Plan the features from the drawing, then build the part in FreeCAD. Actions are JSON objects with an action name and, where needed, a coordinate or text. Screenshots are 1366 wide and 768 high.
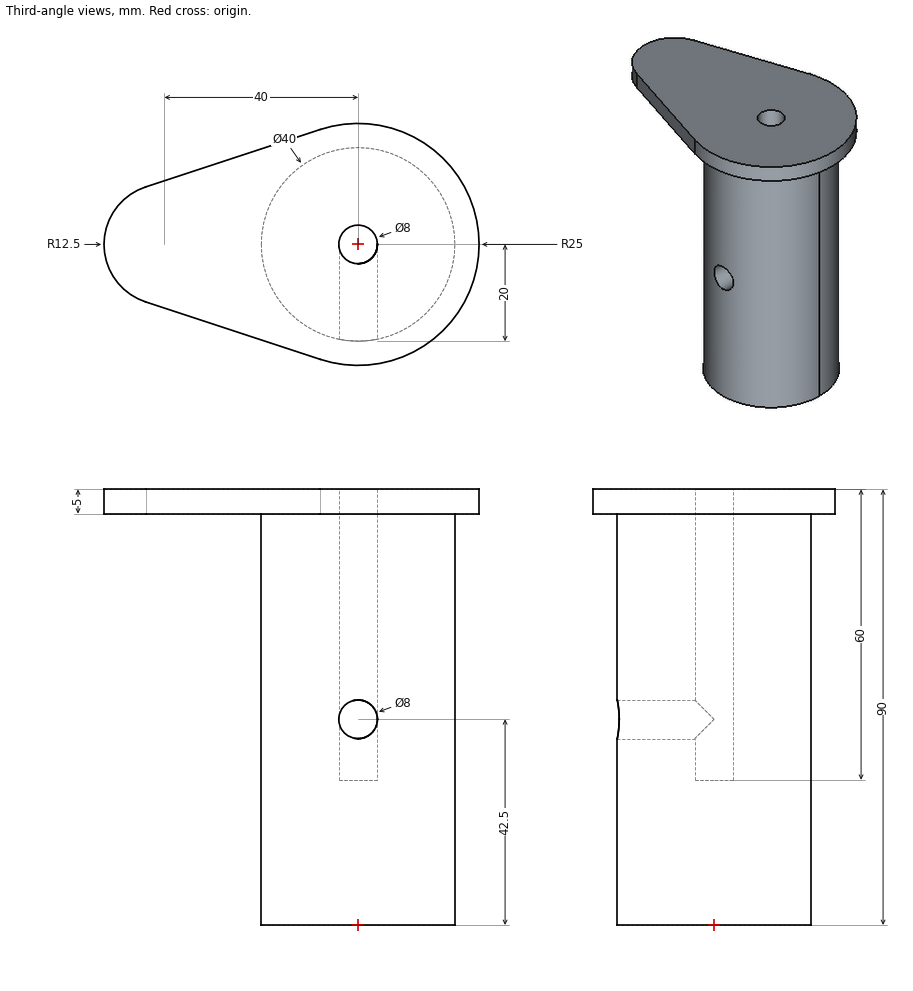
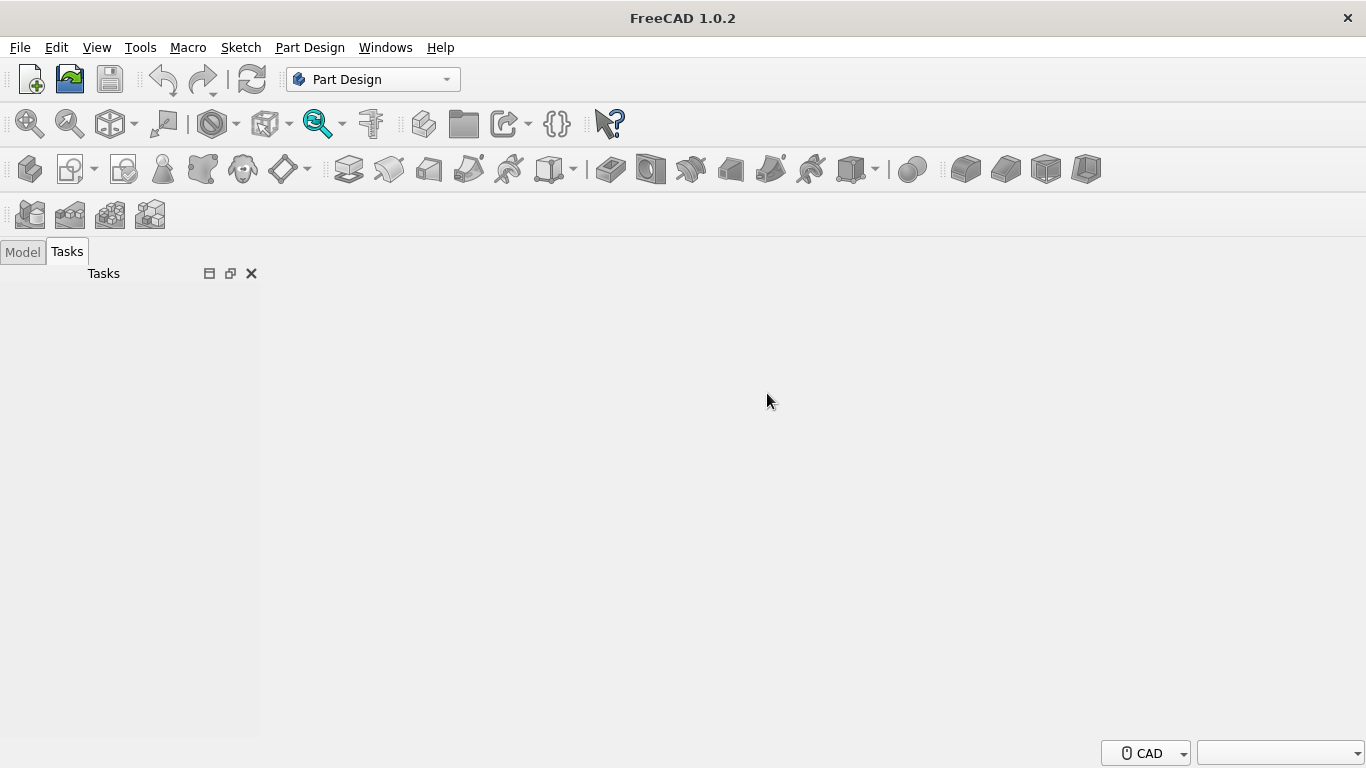
{"action": "key", "text": "ctrl+n"}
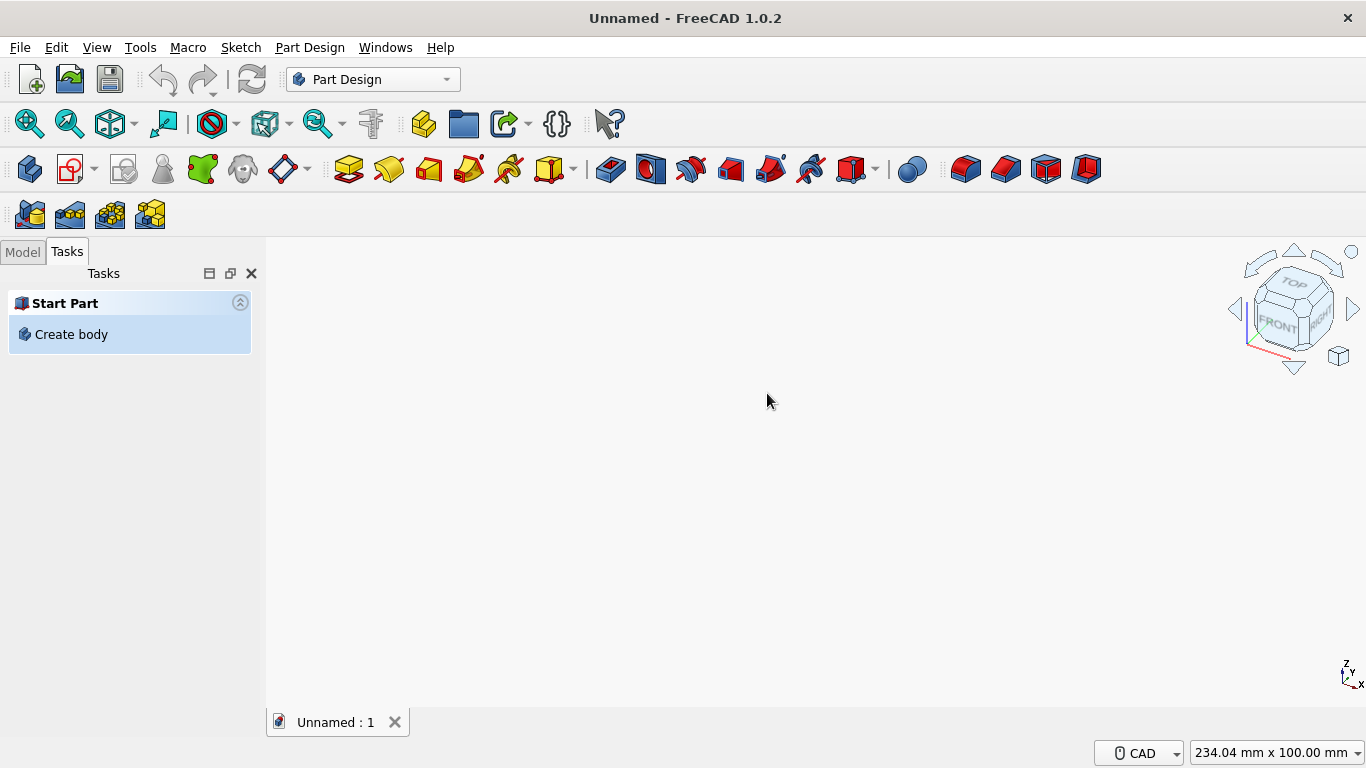
{"action": "left_click", "coordinate": [70, 170]}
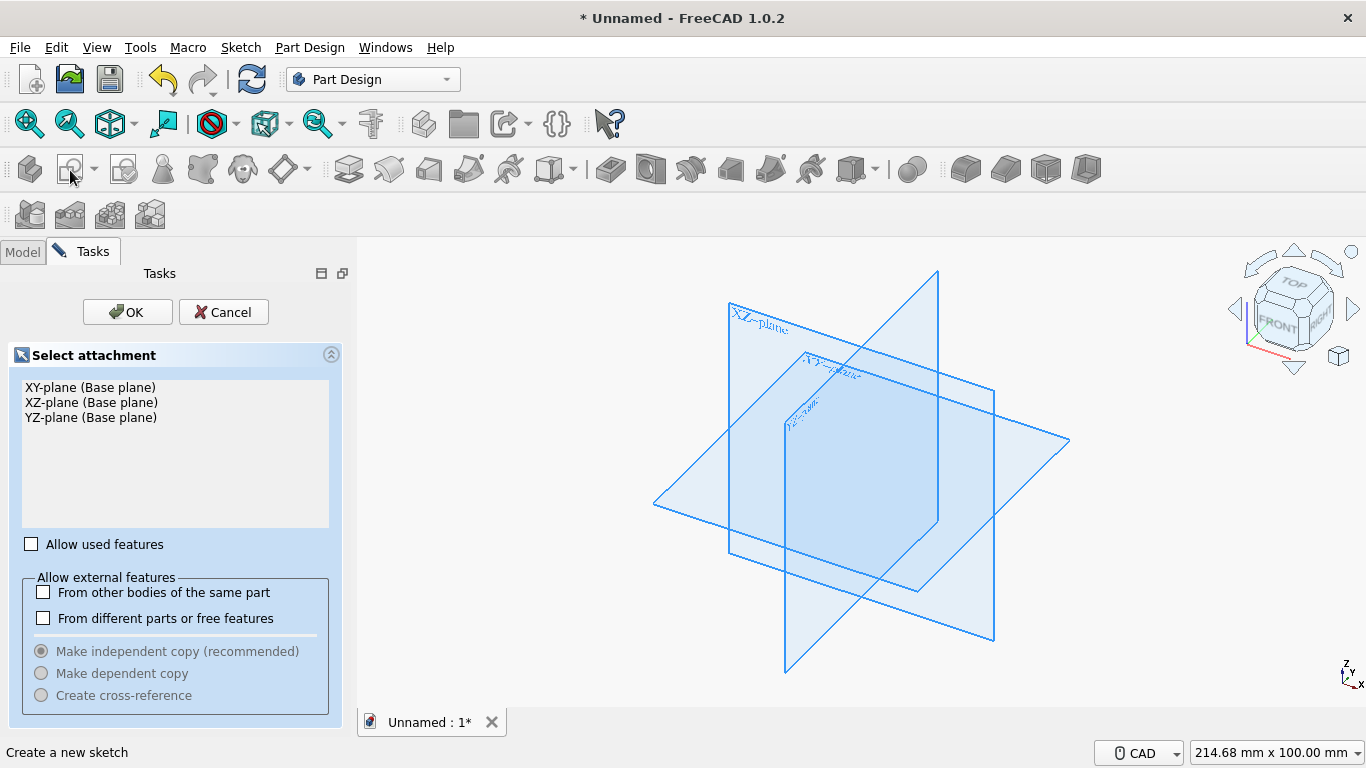
{"action": "left_click", "coordinate": [82, 388]}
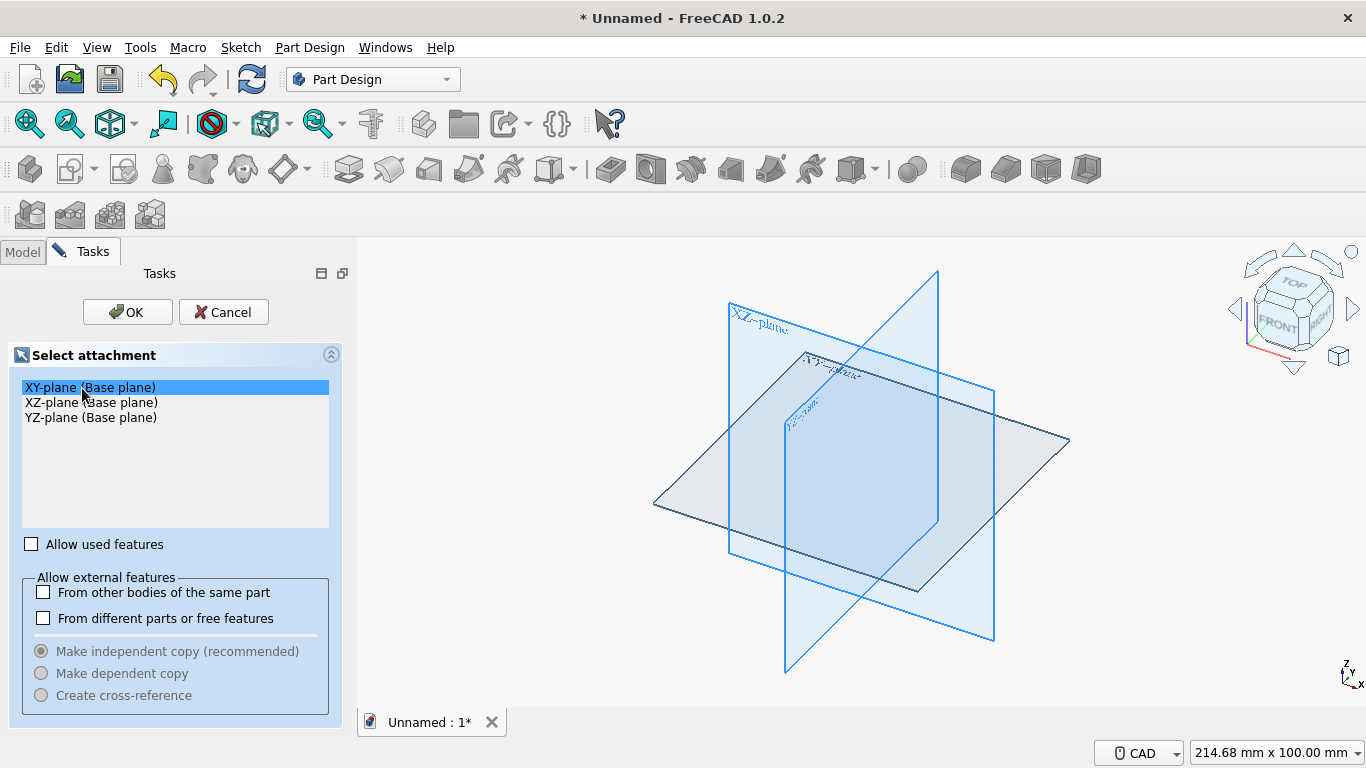
{"action": "left_click", "coordinate": [128, 312]}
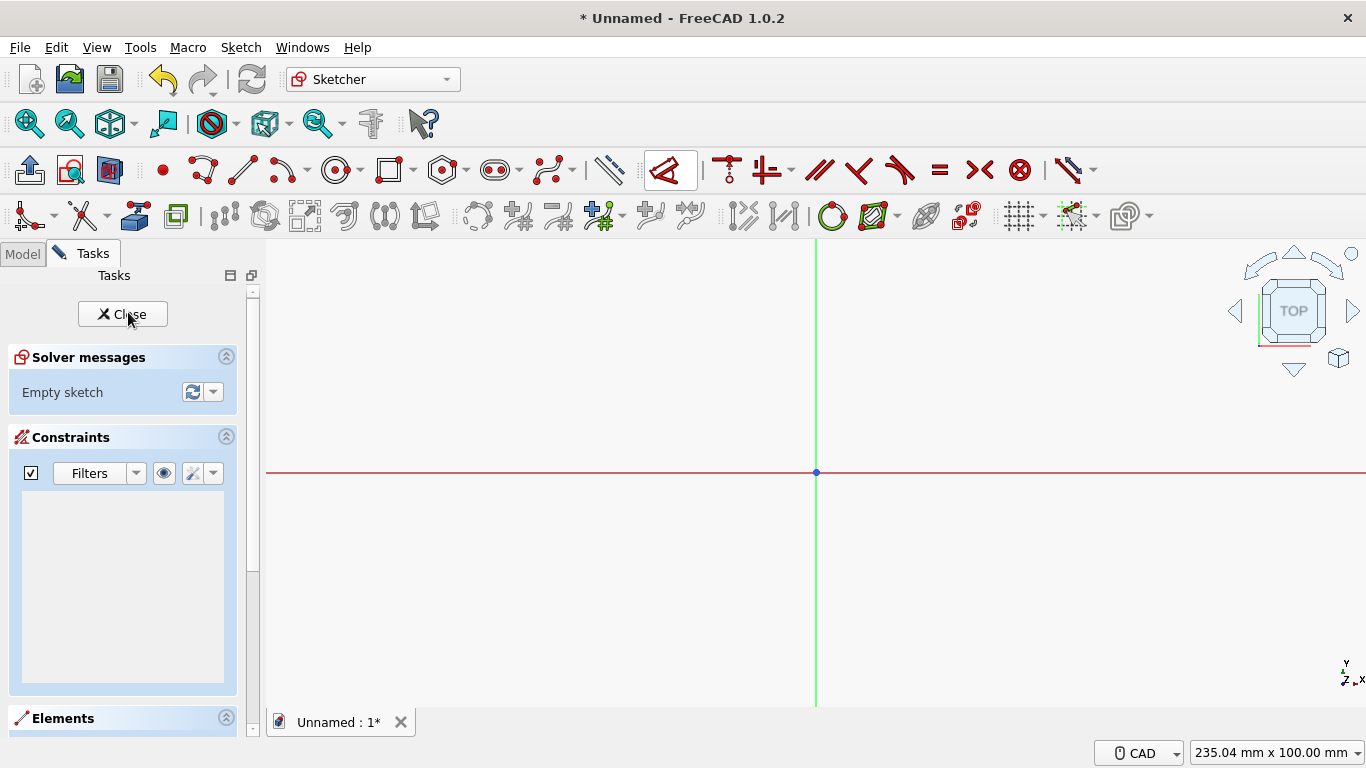
{"action": "scroll", "coordinate": [955, 473], "scroll_direction": "up", "scroll_amount": 2}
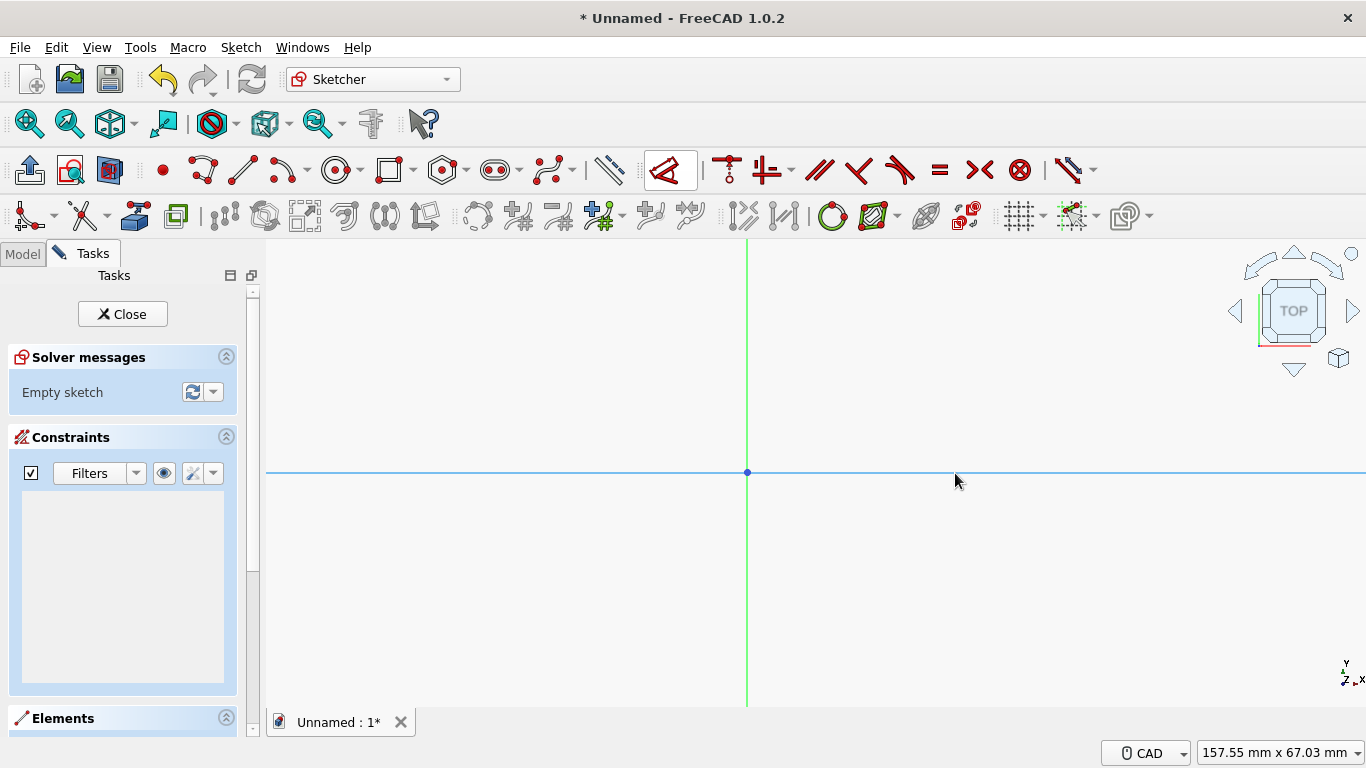
{"action": "key", "text": "g c"}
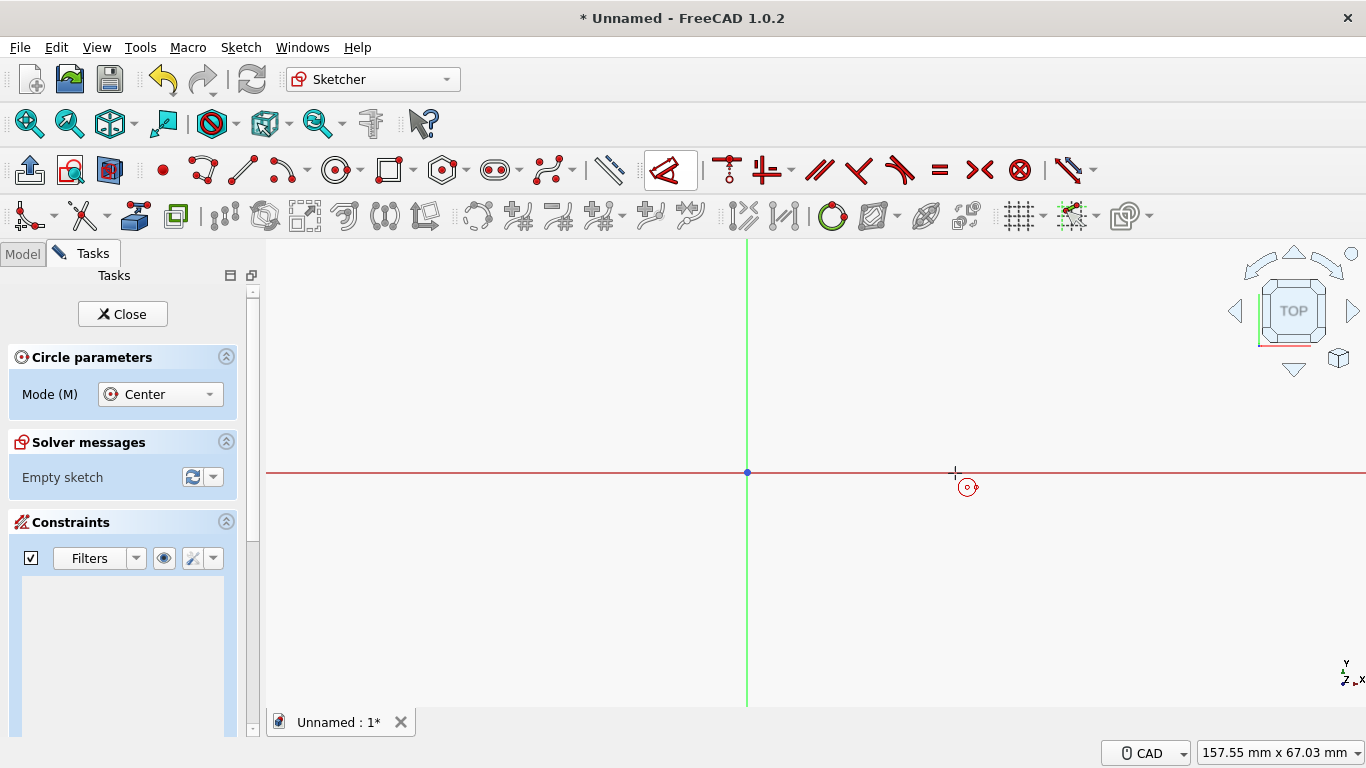
{"action": "left_click", "coordinate": [747, 473]}
{"action": "mouse_move", "coordinate": [846, 374]}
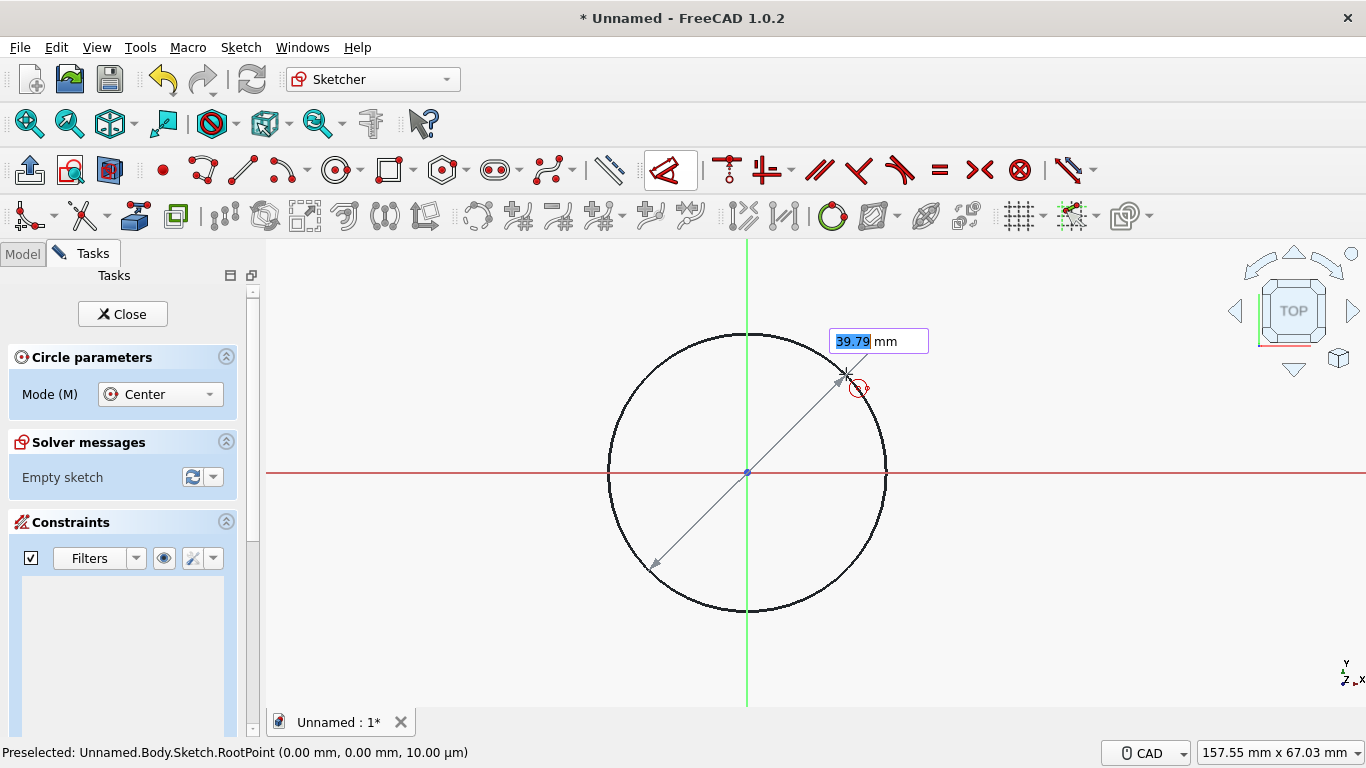
{"action": "type", "text": "40"}
{"action": "key", "text": "Return"}
{"action": "key", "text": "Escape"}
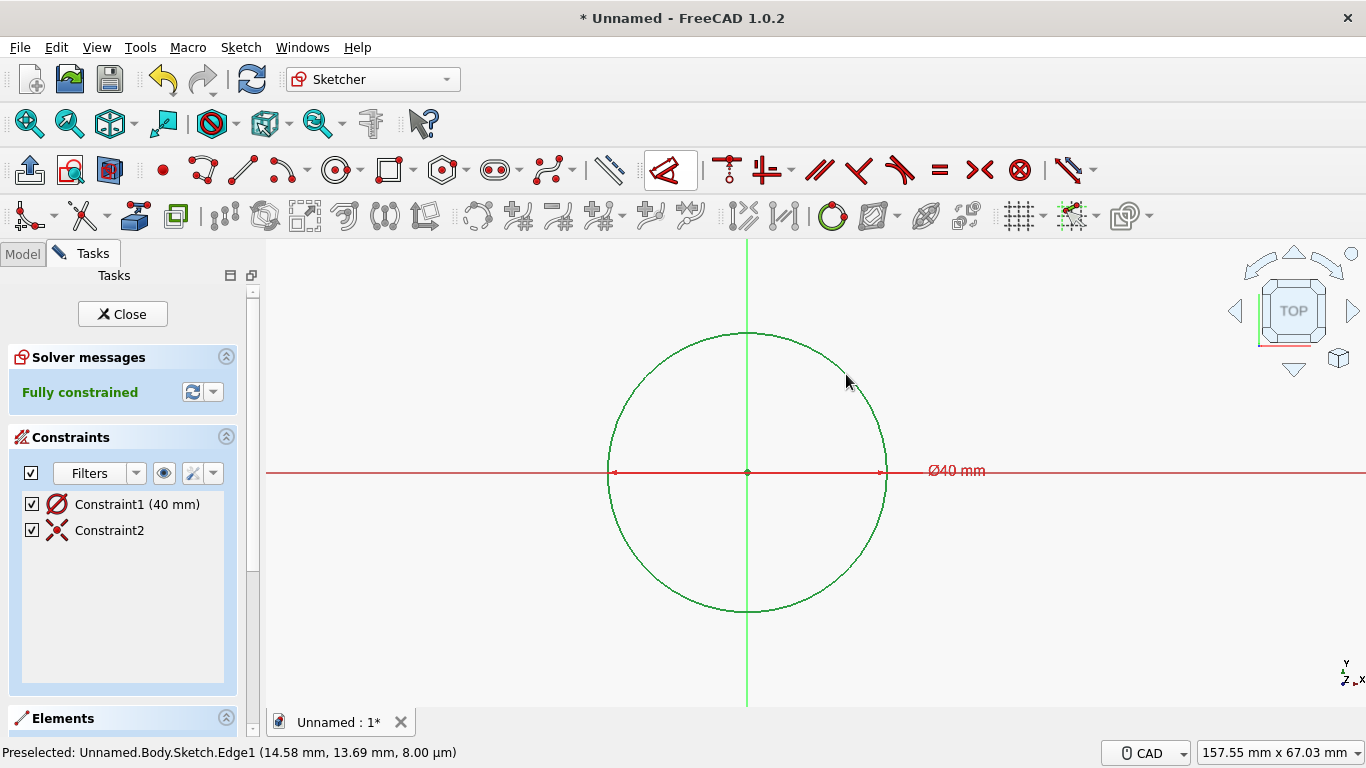
{"action": "left_click", "coordinate": [123, 314]}